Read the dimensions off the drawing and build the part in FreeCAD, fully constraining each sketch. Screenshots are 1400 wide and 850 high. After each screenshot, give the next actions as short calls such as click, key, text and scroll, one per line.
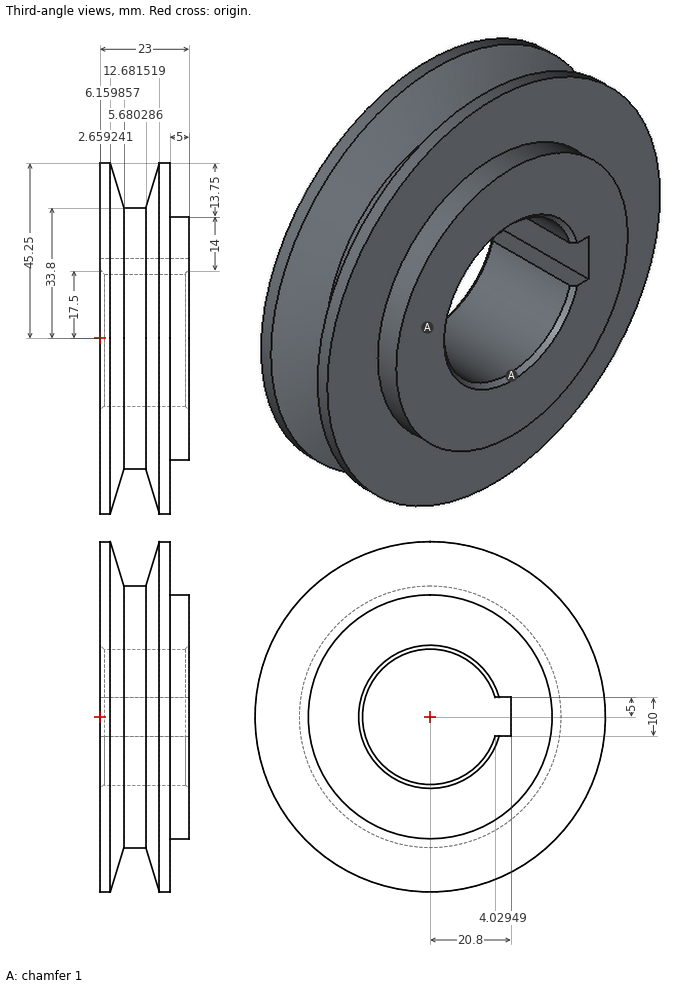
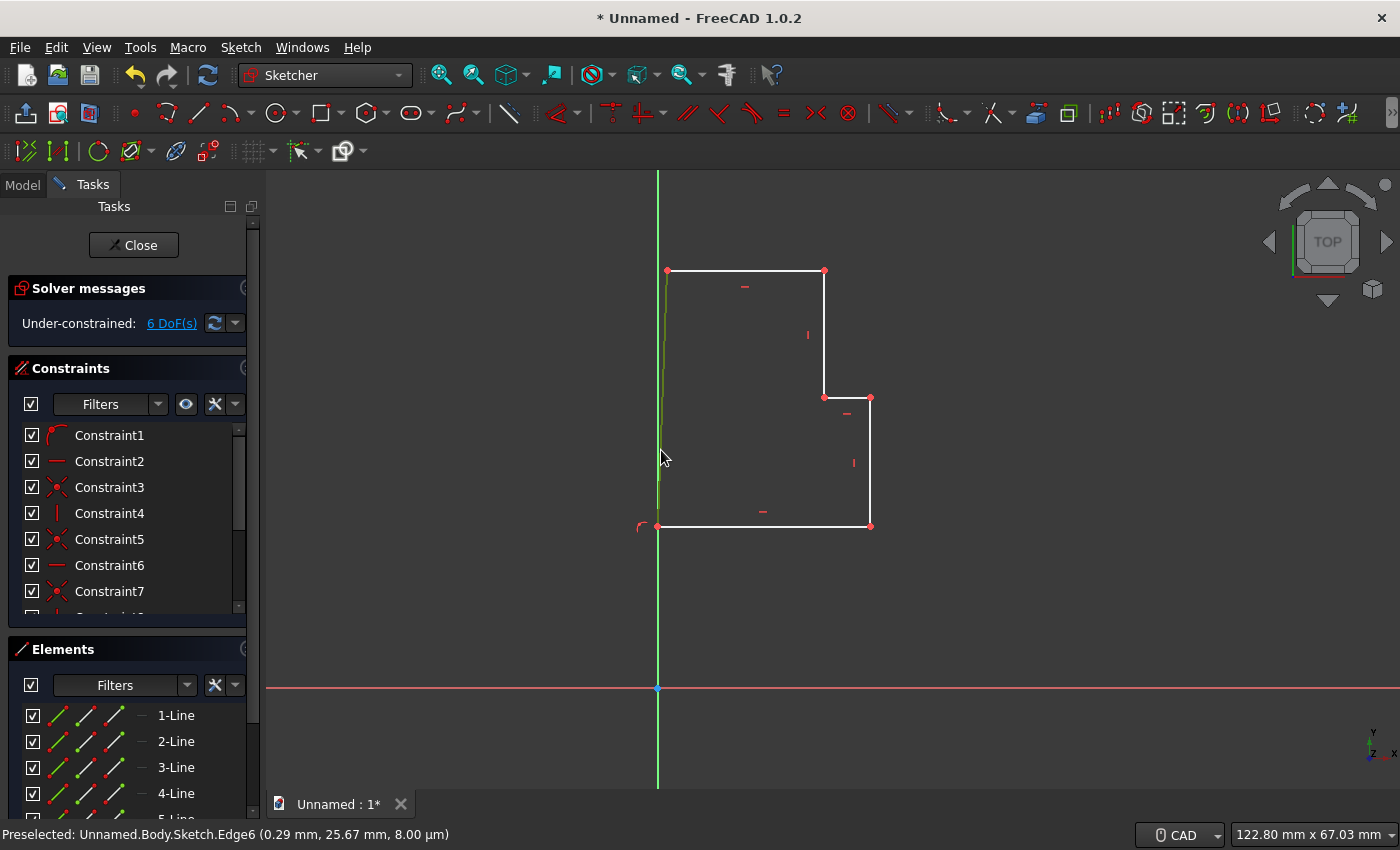
key(v)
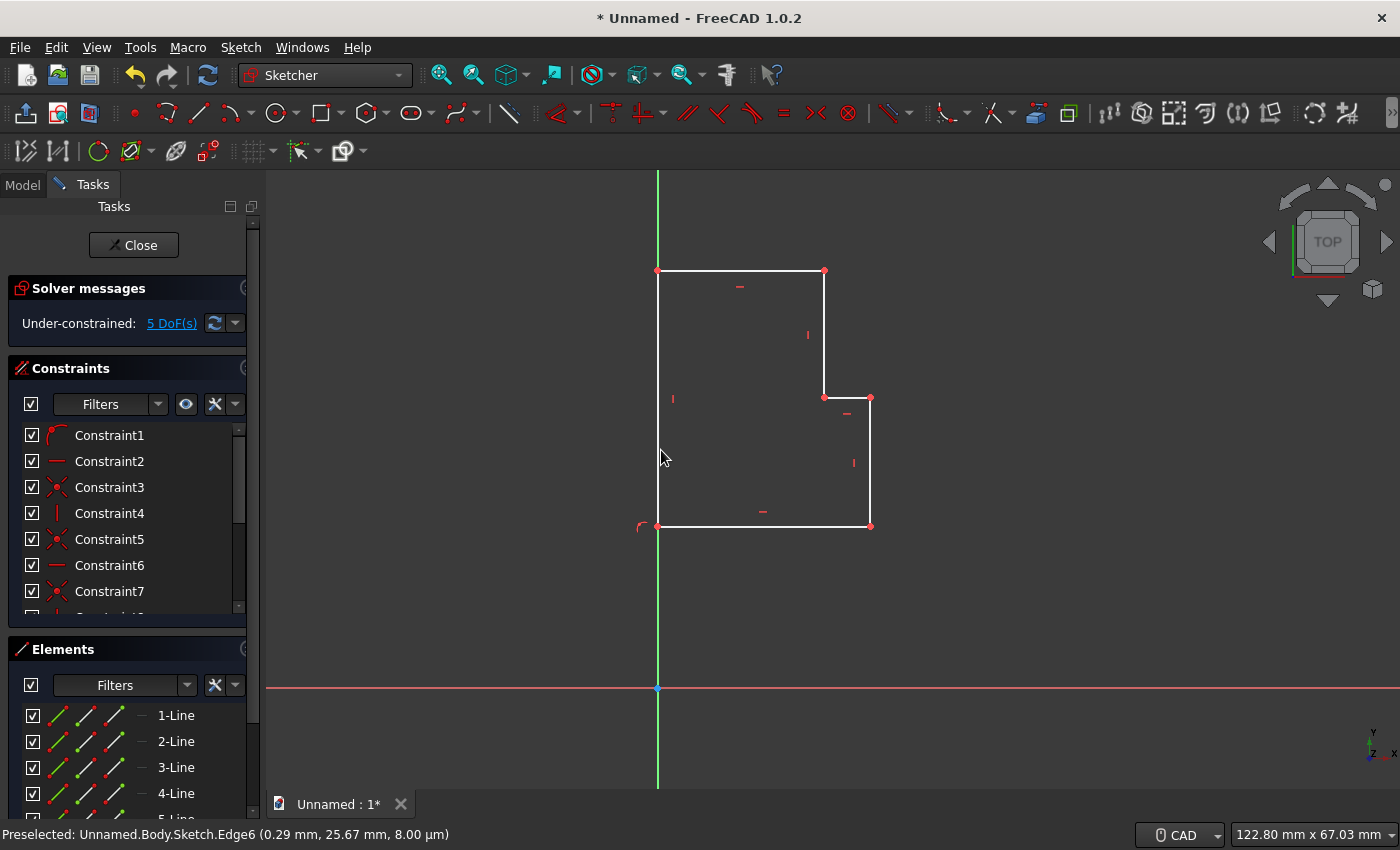
key(d)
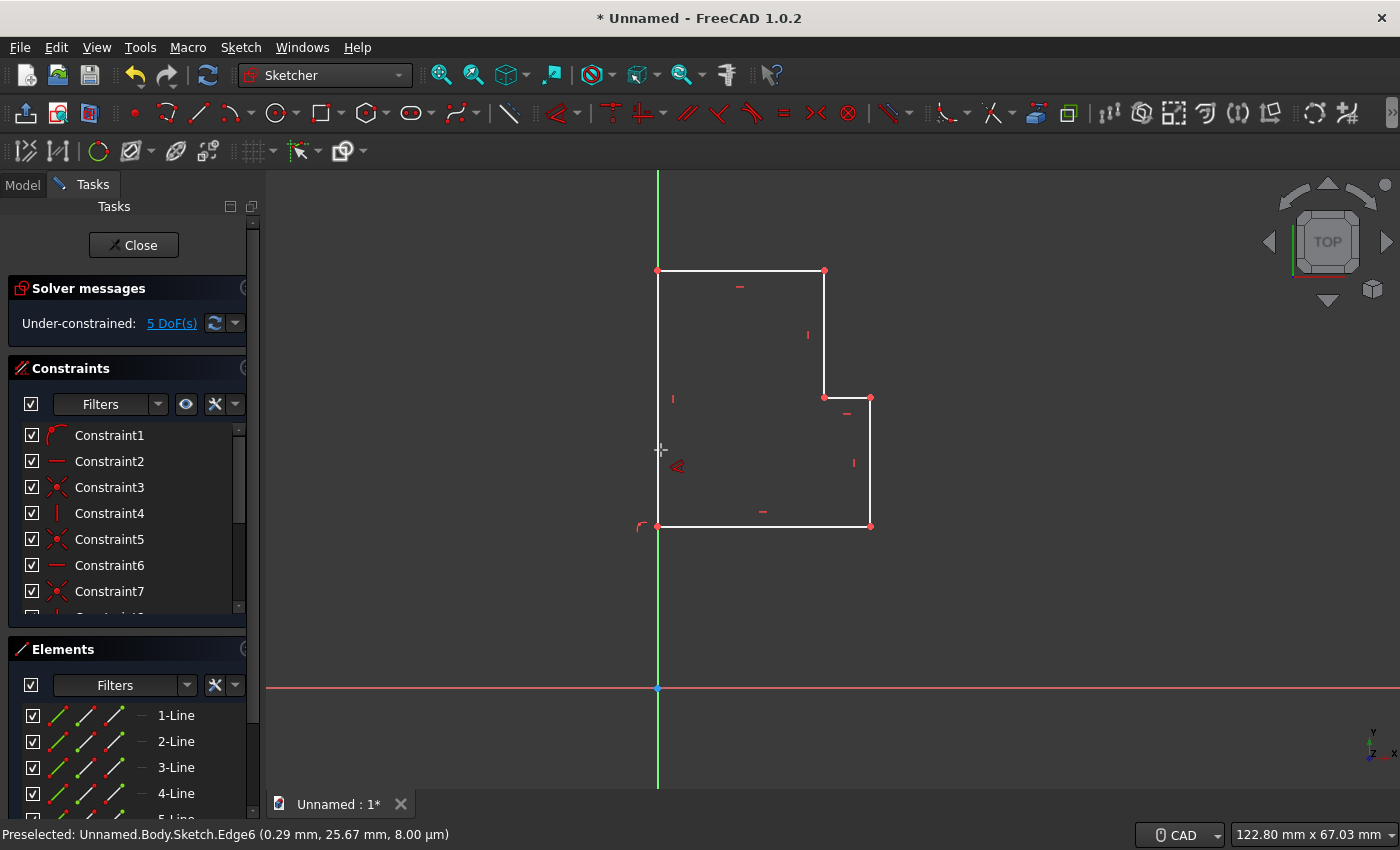
click(856, 398)
click(847, 364)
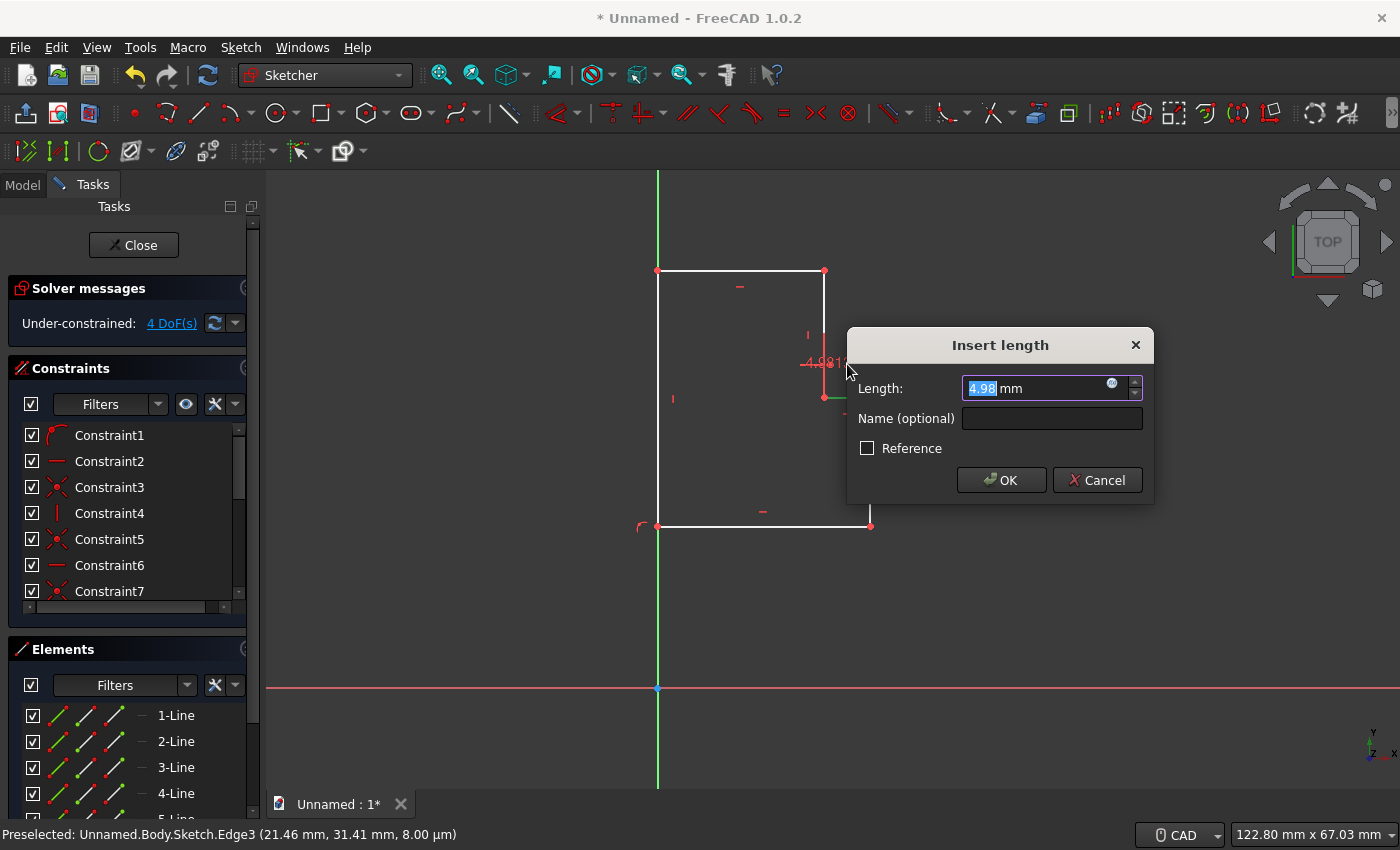
text(5)
key(Return)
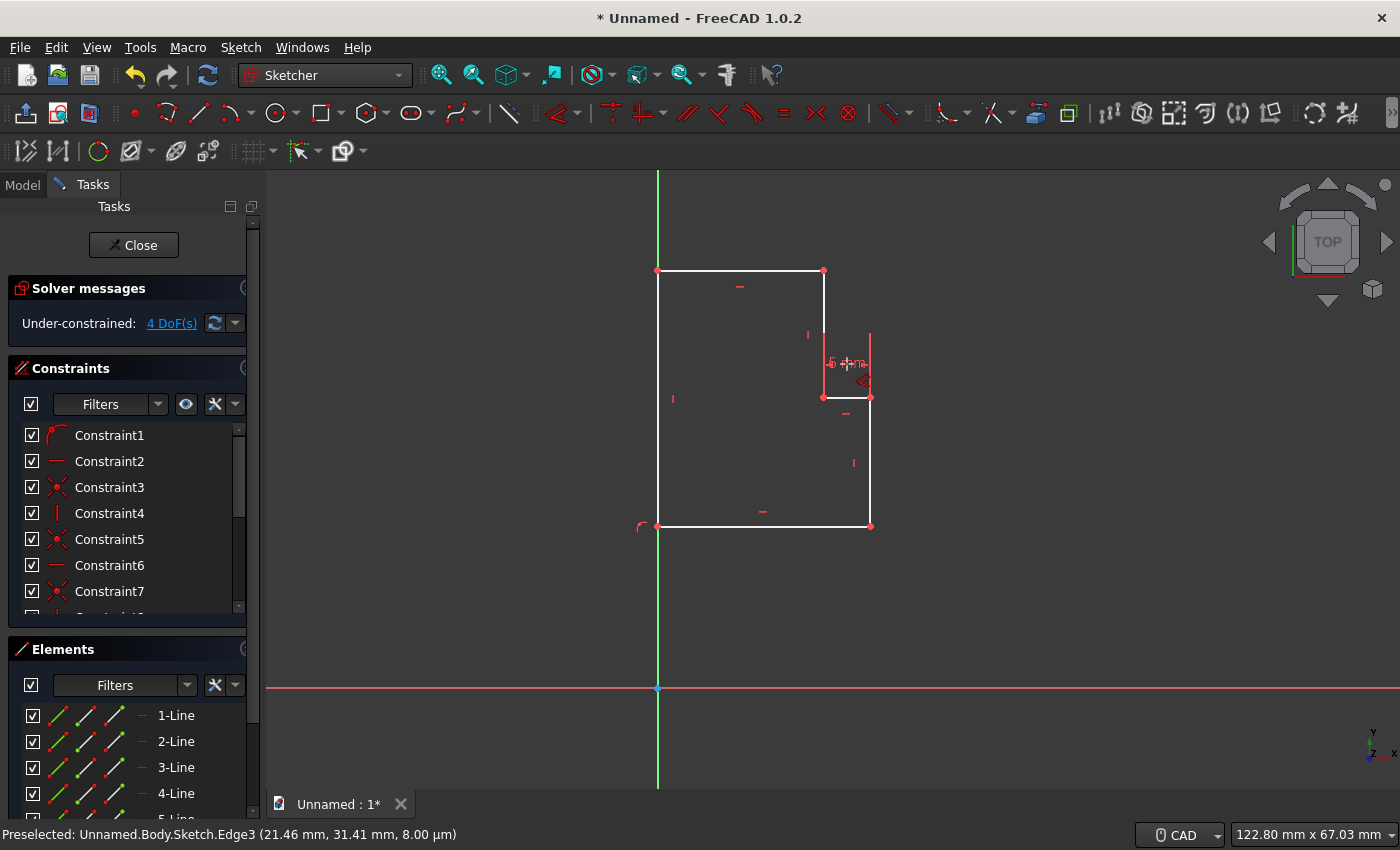
click(722, 527)
click(764, 561)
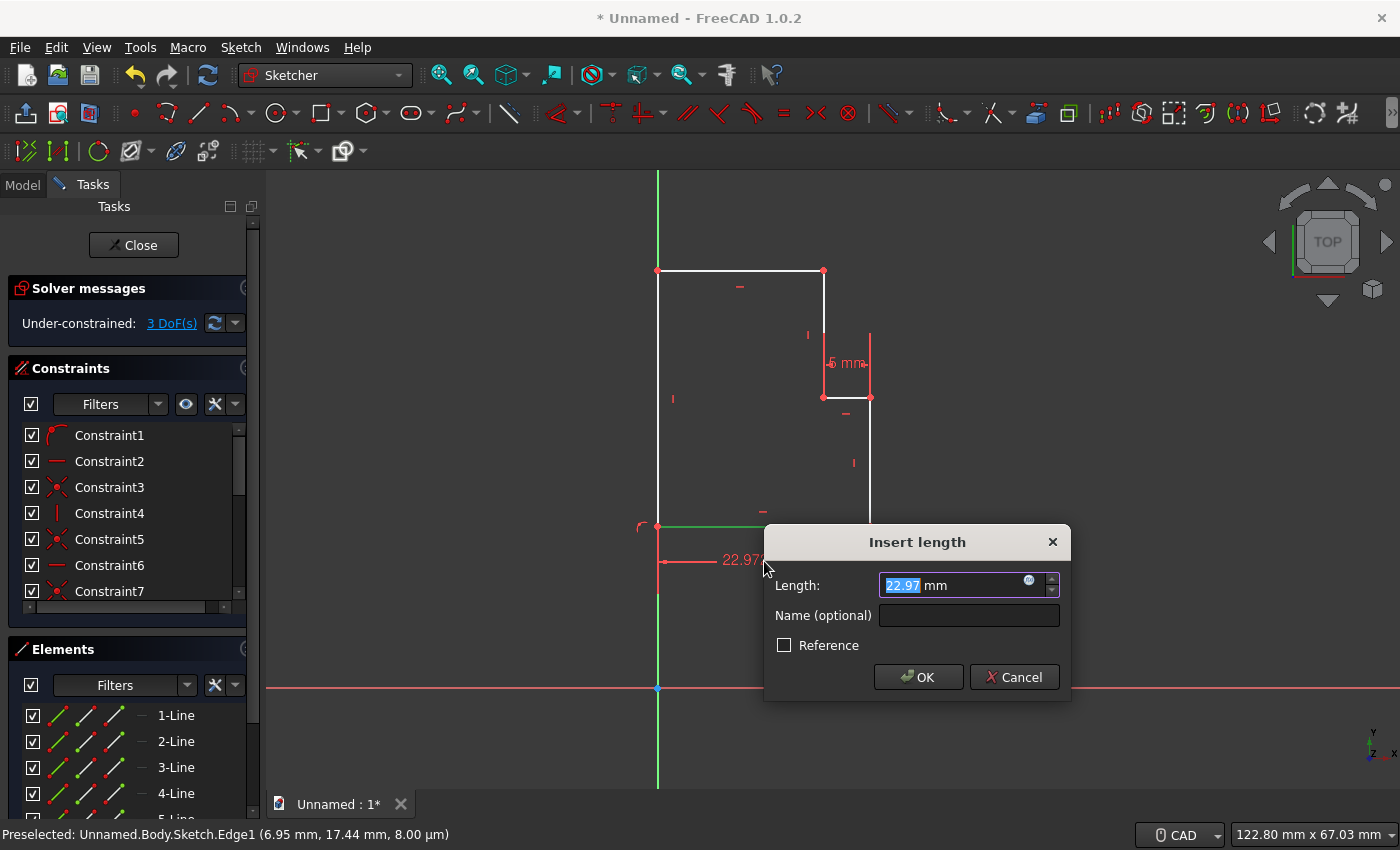
text(23)
key(Return)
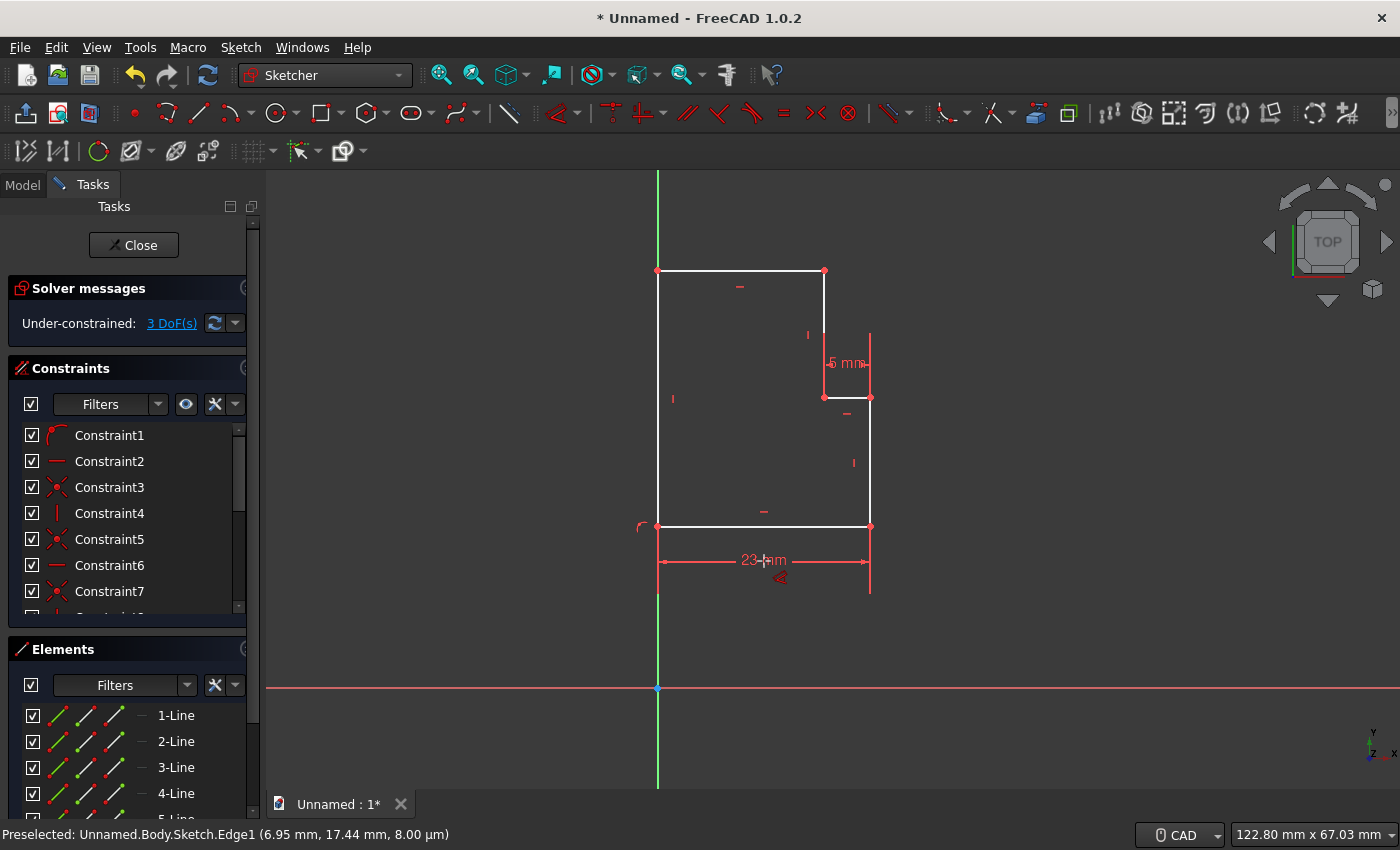
click(870, 488)
click(904, 462)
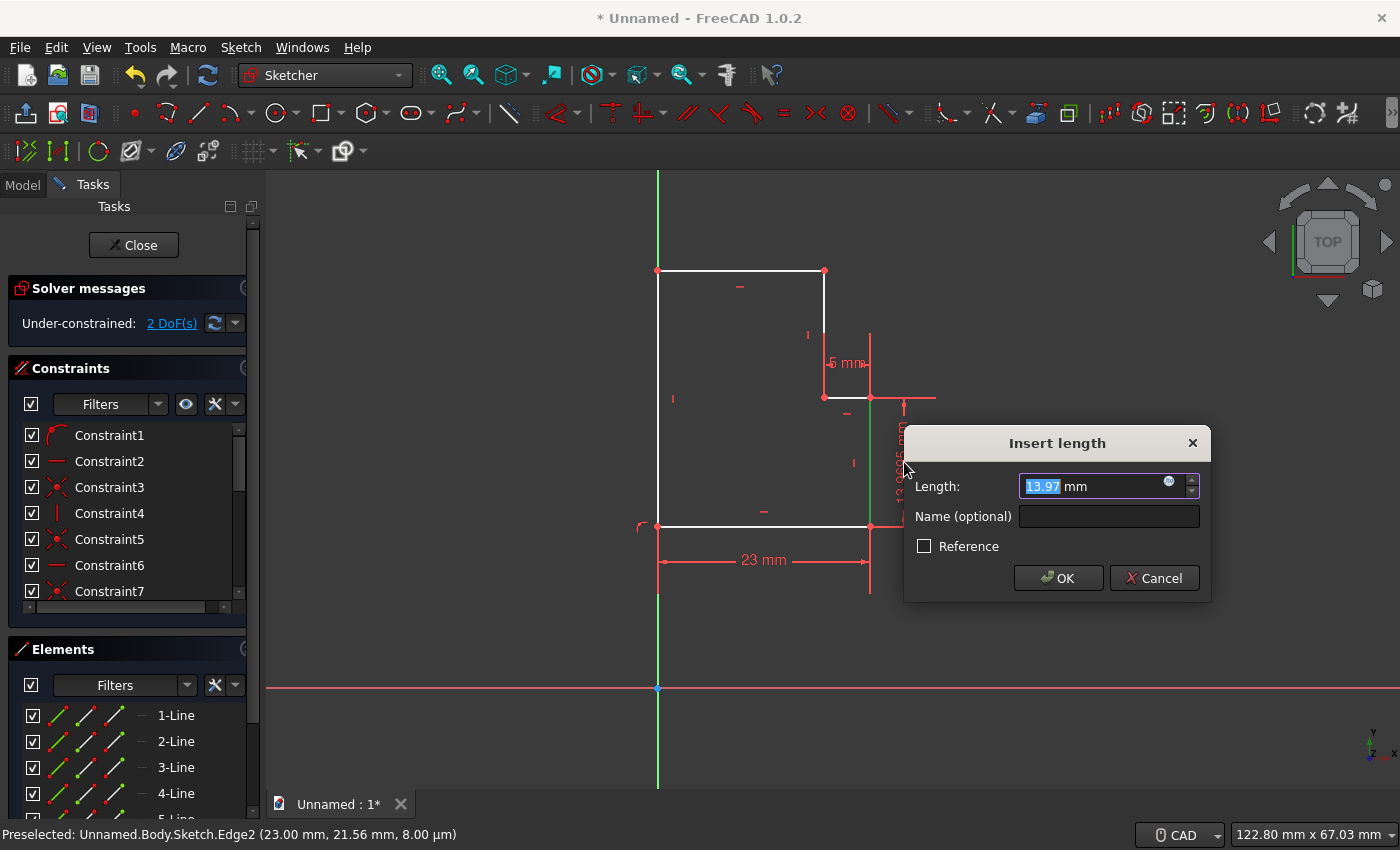
text(14)
key(Return)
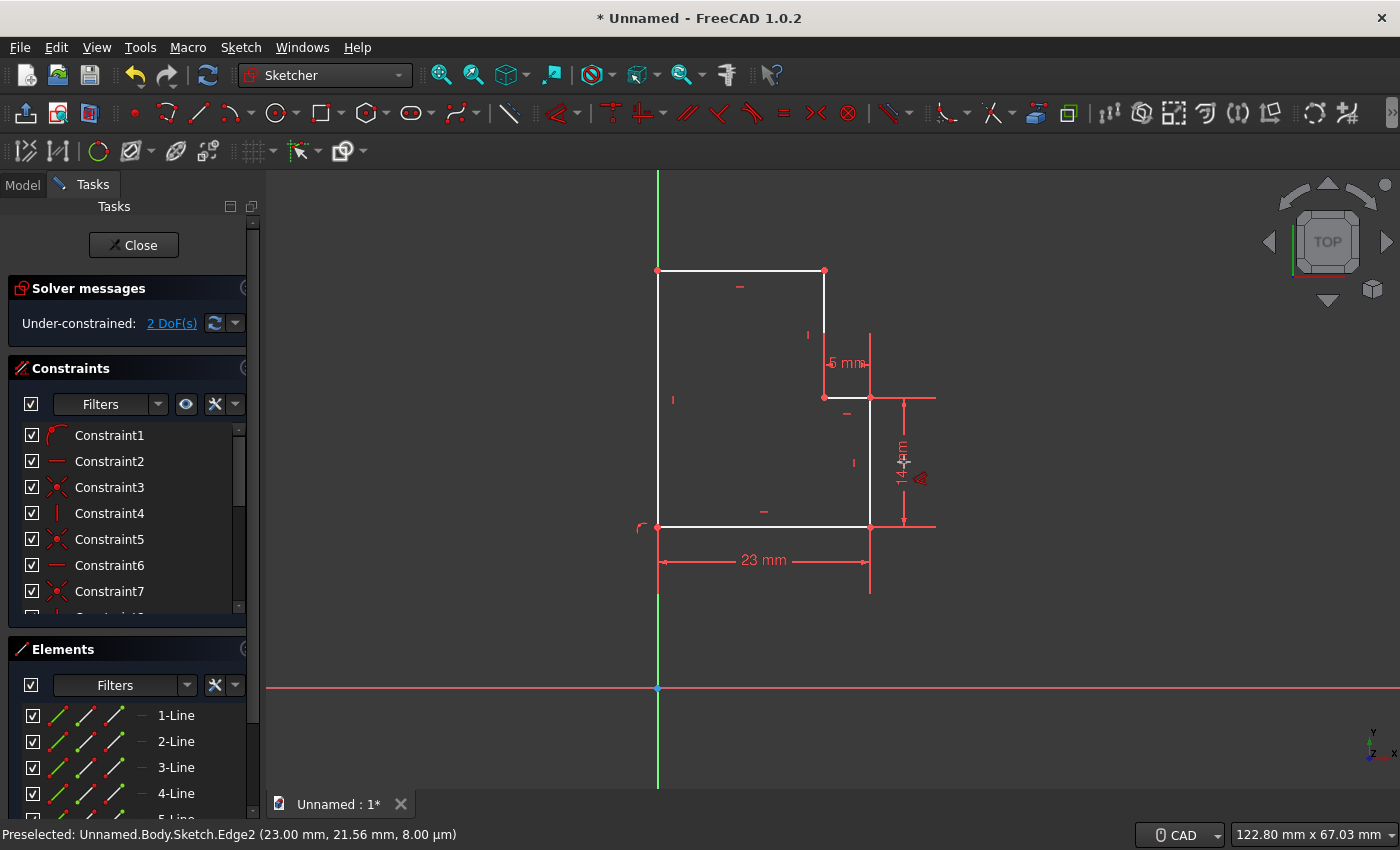
click(824, 360)
click(858, 334)